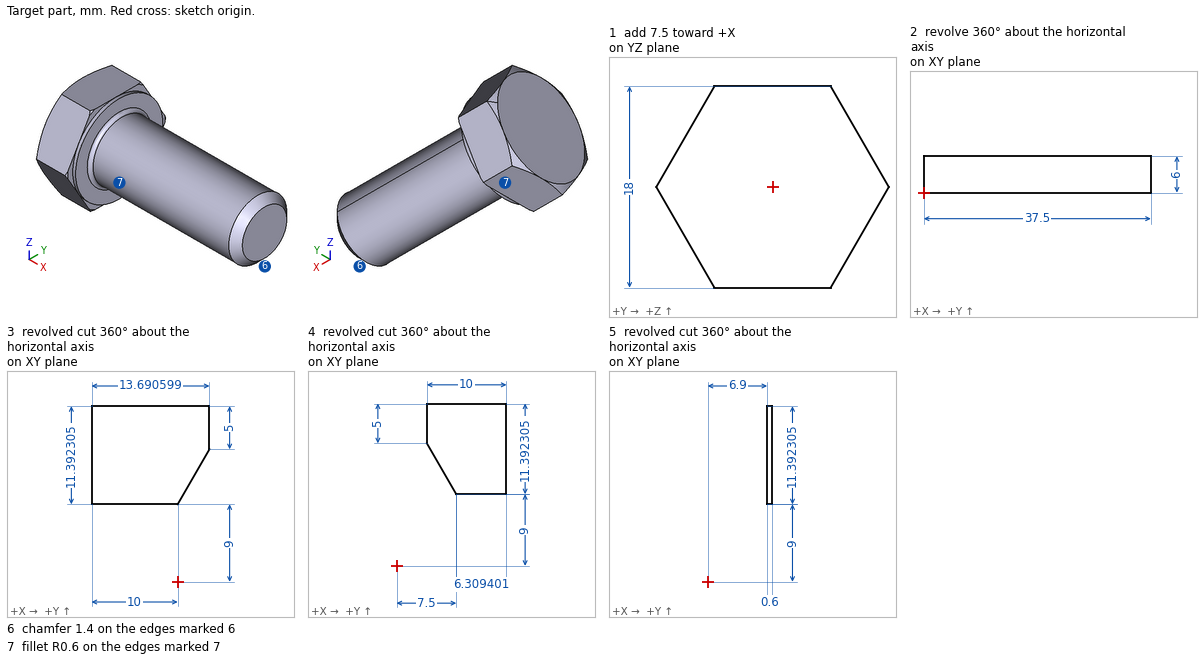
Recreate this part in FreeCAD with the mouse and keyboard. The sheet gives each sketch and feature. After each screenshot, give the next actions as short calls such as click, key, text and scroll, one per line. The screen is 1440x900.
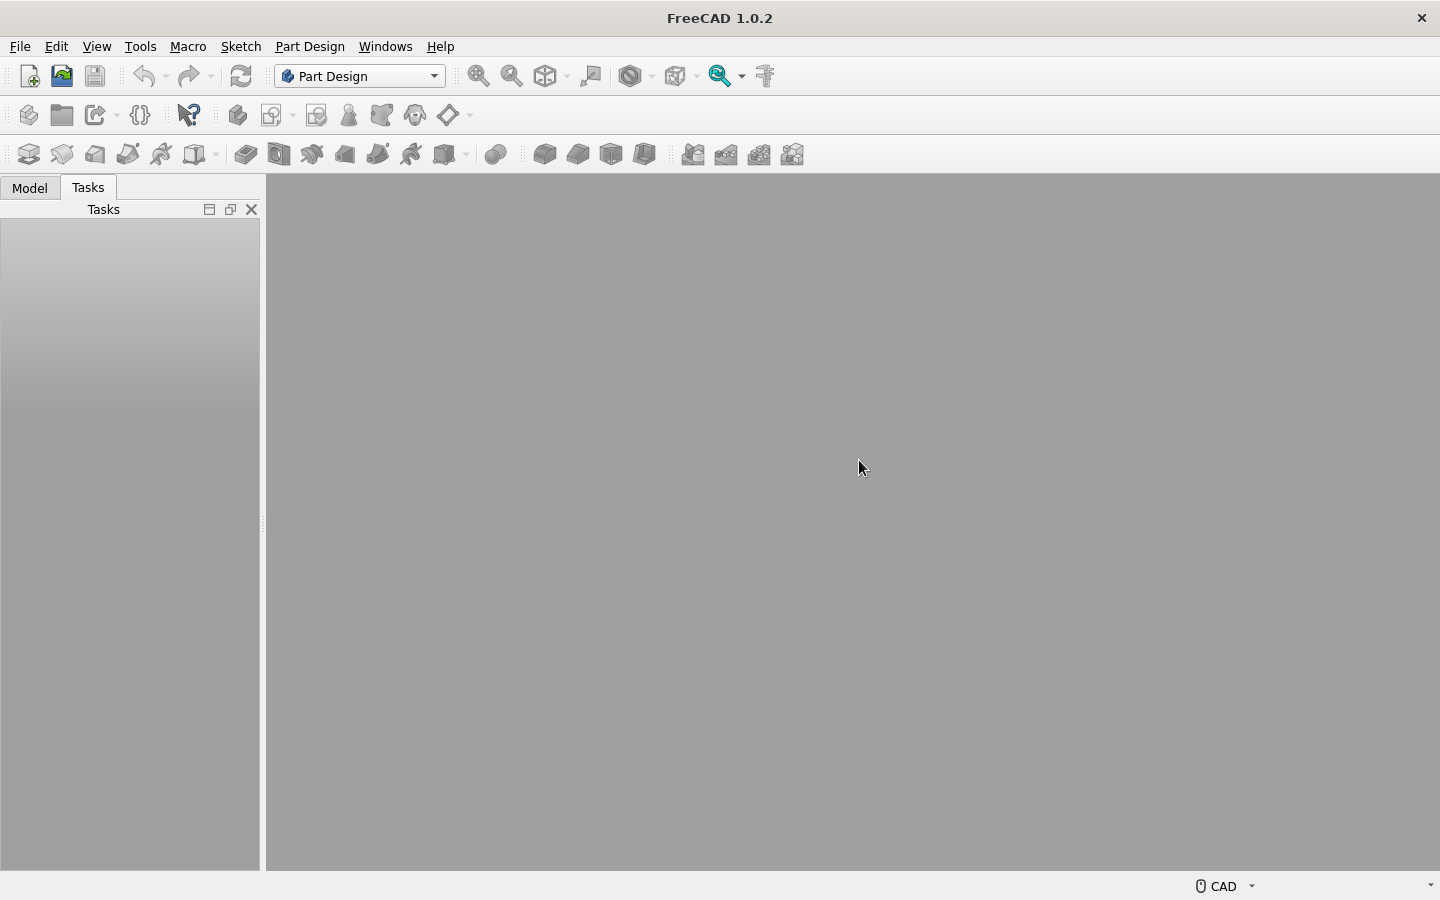
key(ctrl+n)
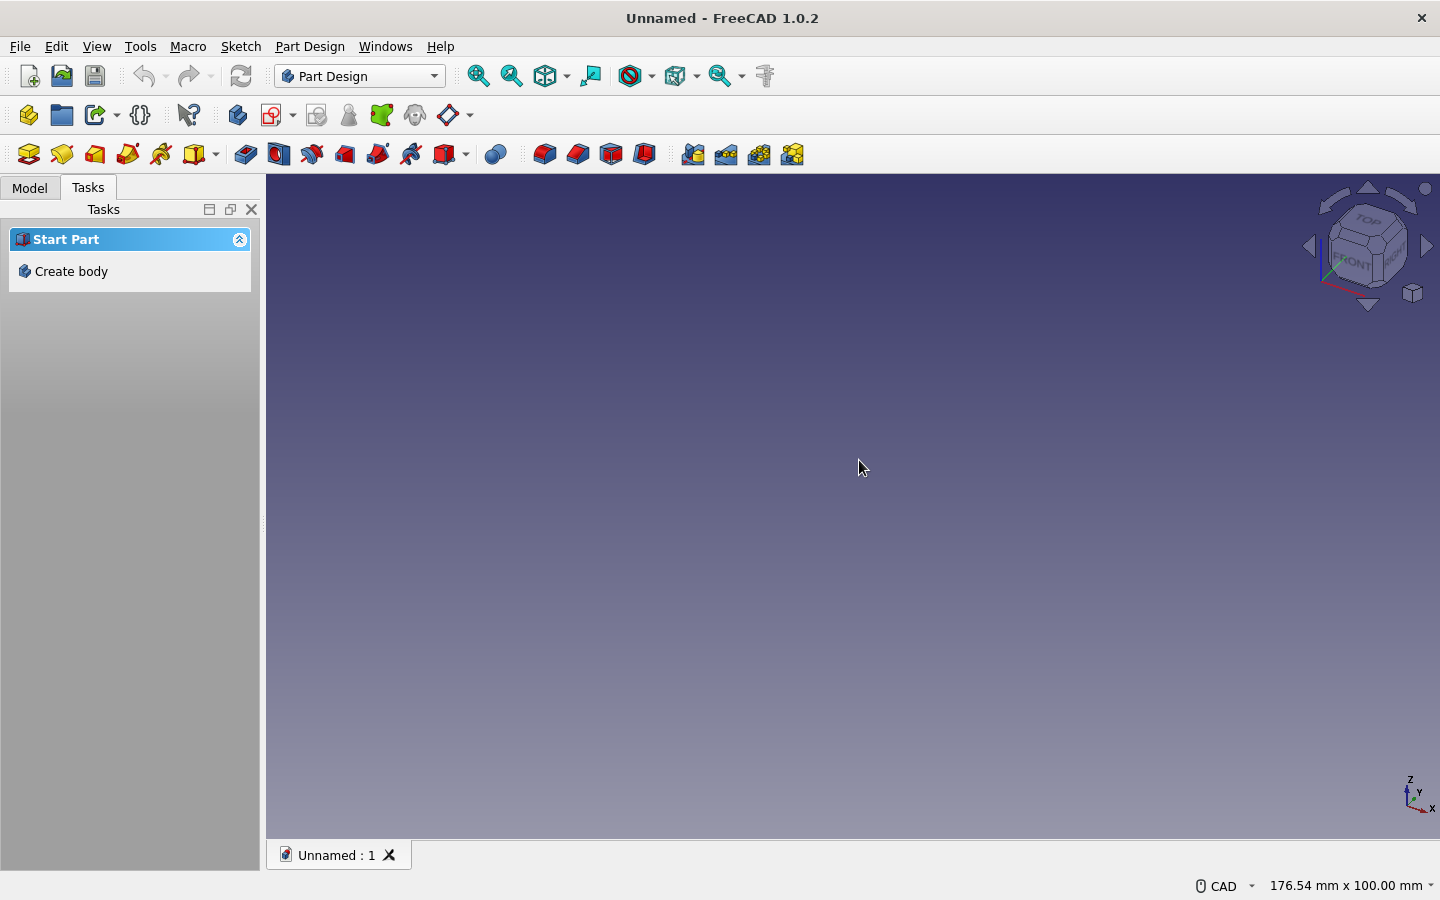
click(270, 116)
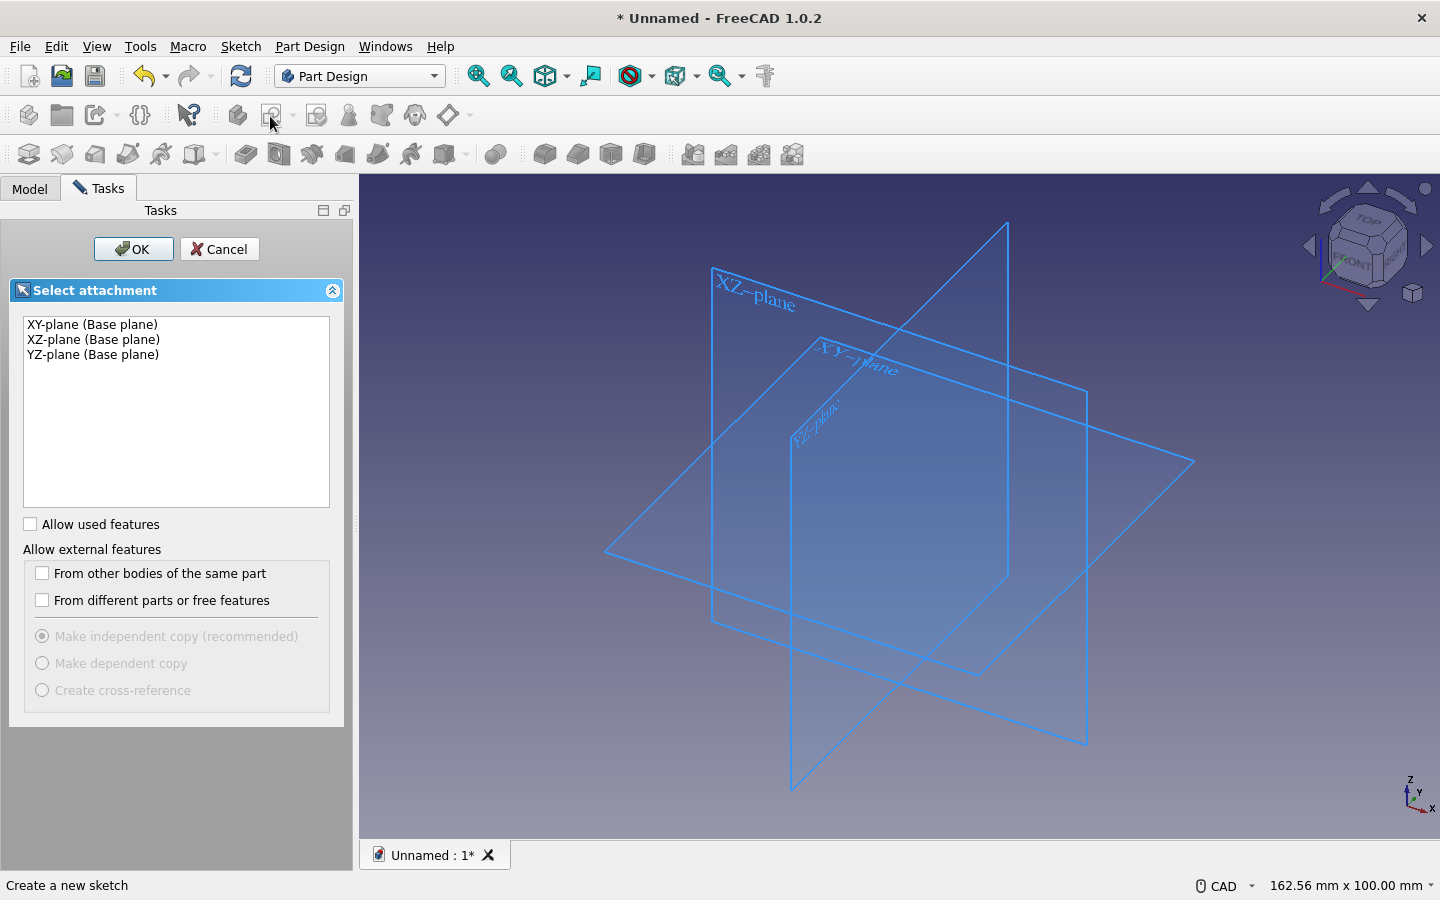
click(84, 354)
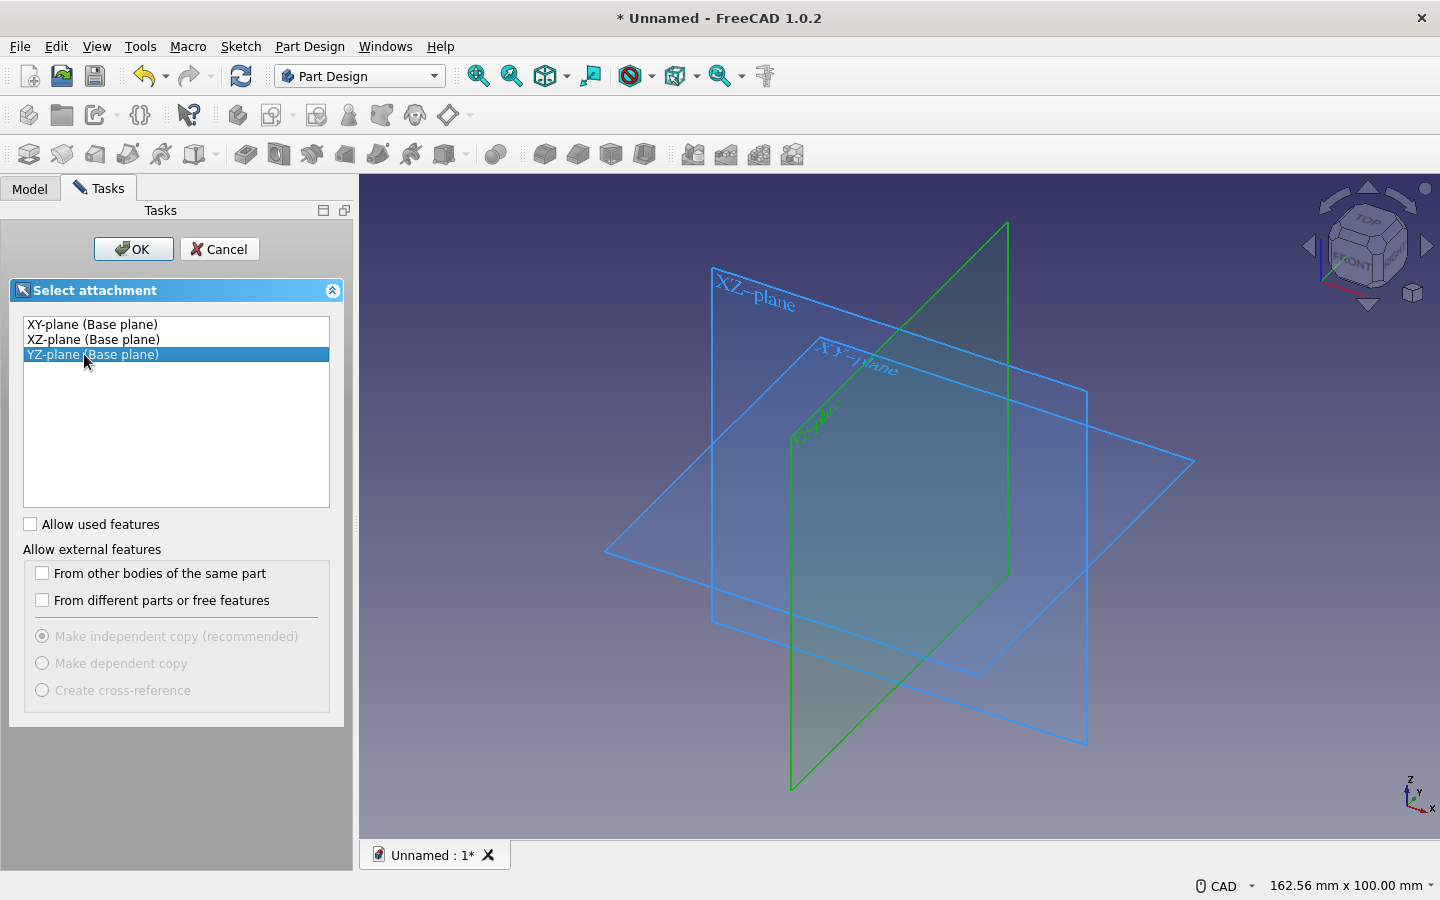
click(134, 249)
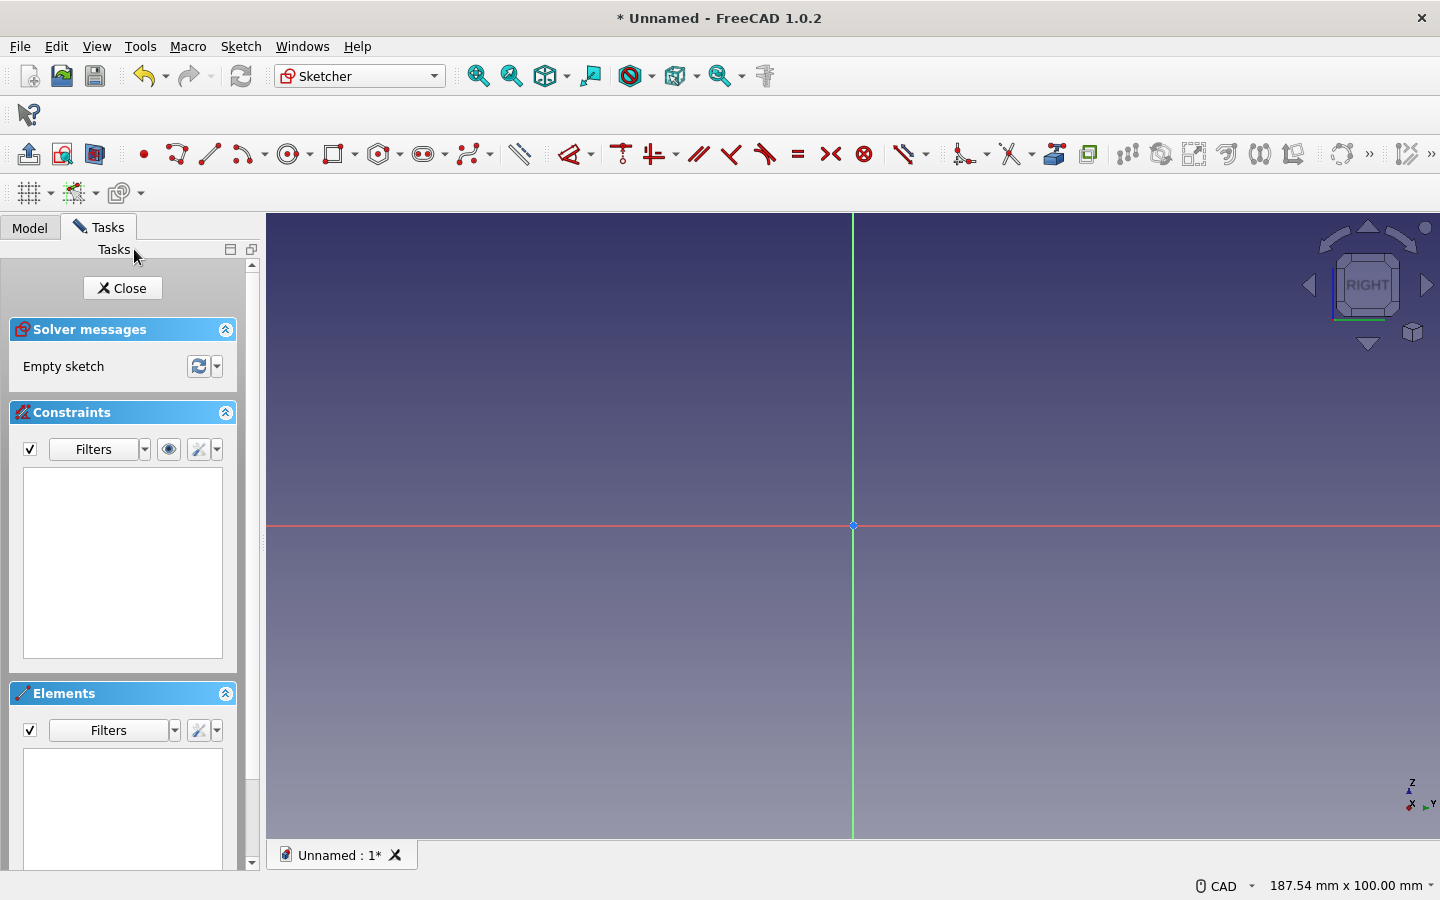
scroll(883, 526, up, 6)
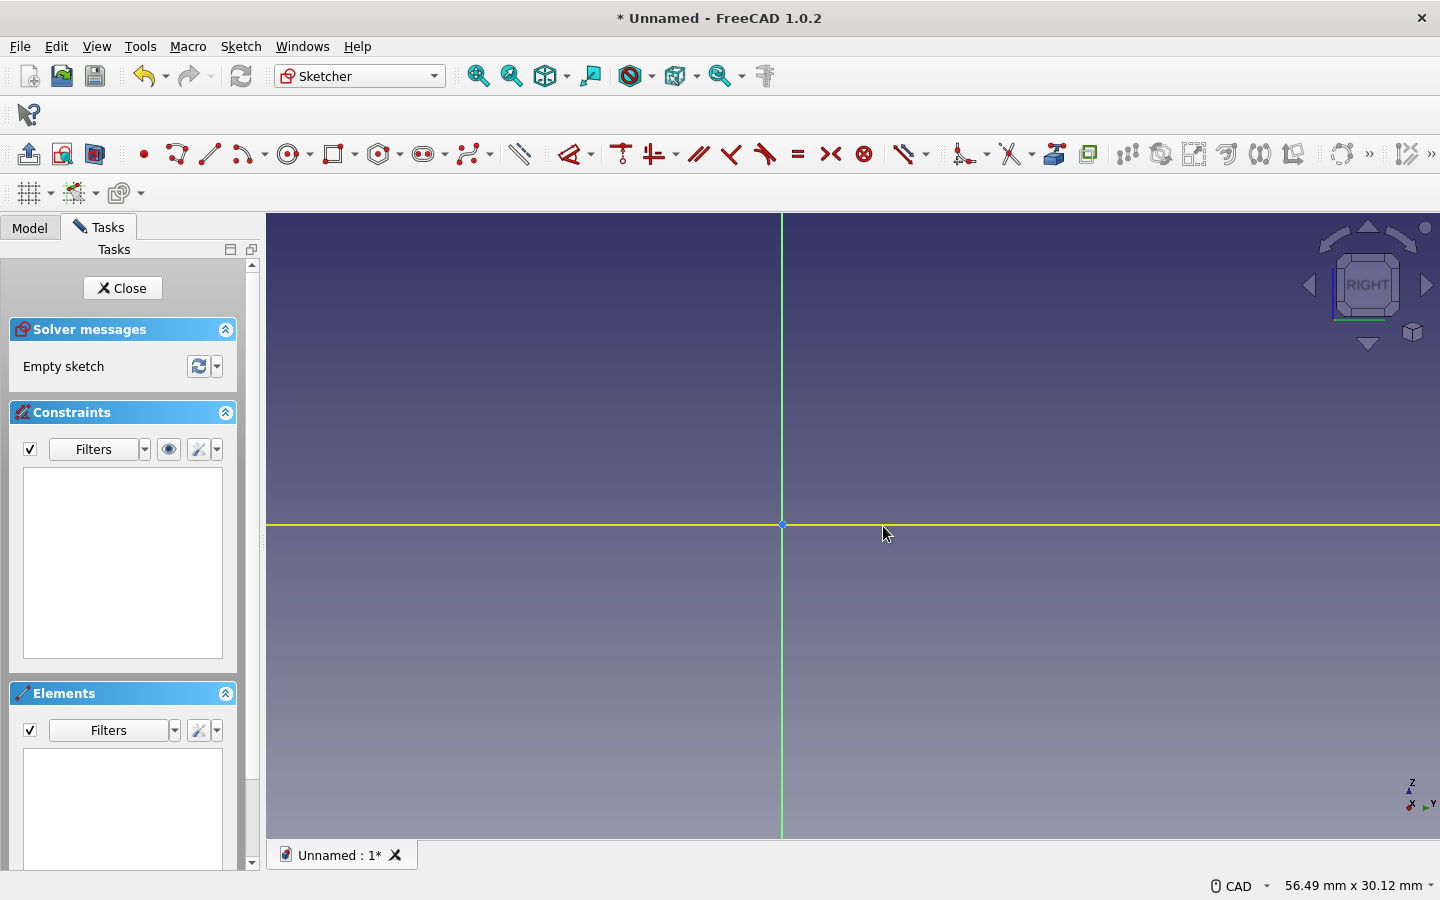
key(g)
key(p)
key(6)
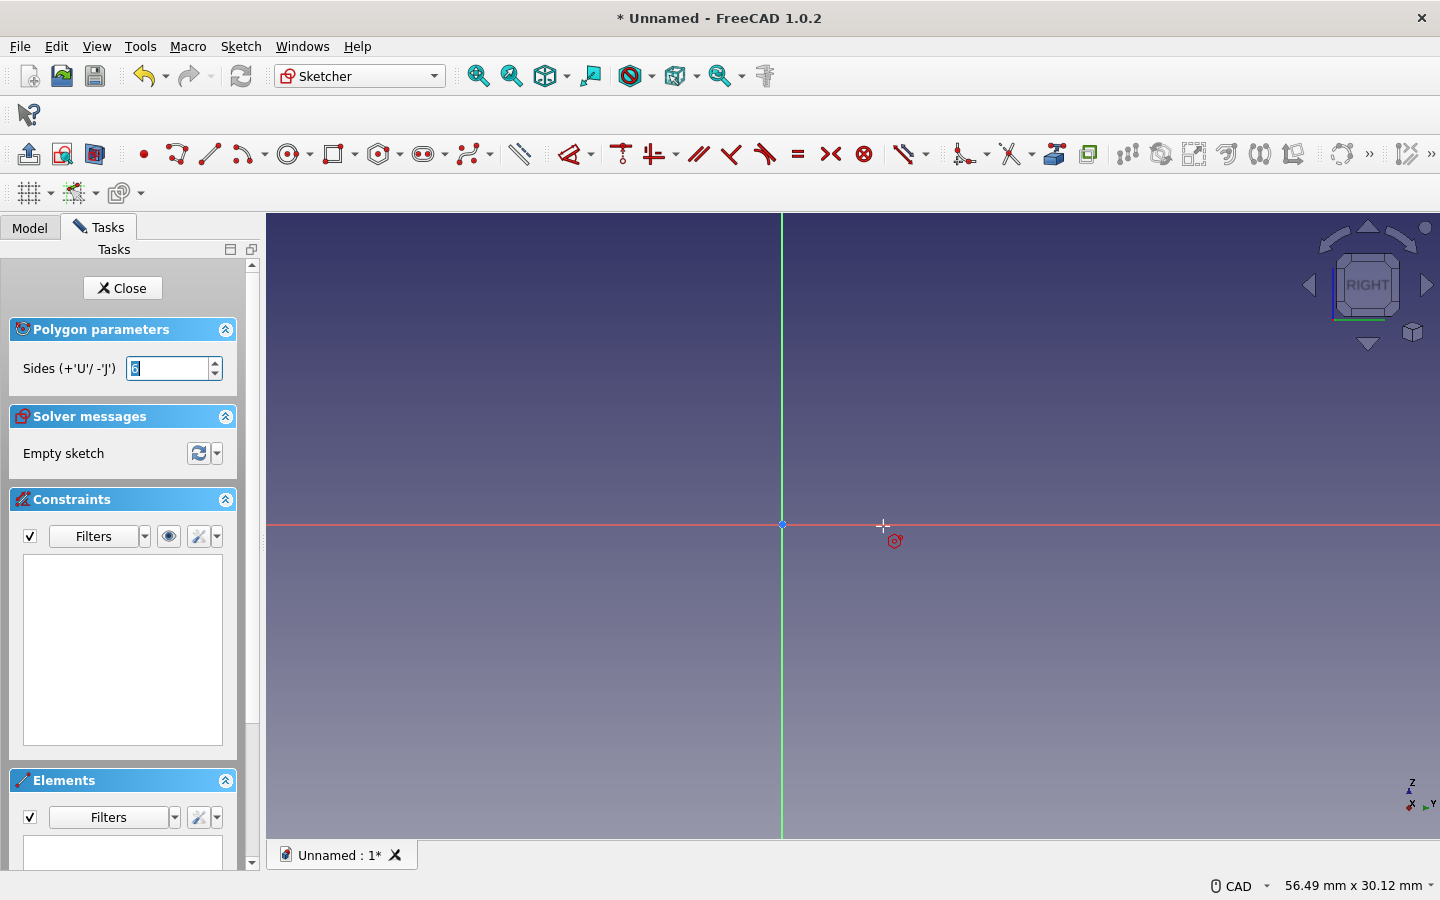
click(782, 525)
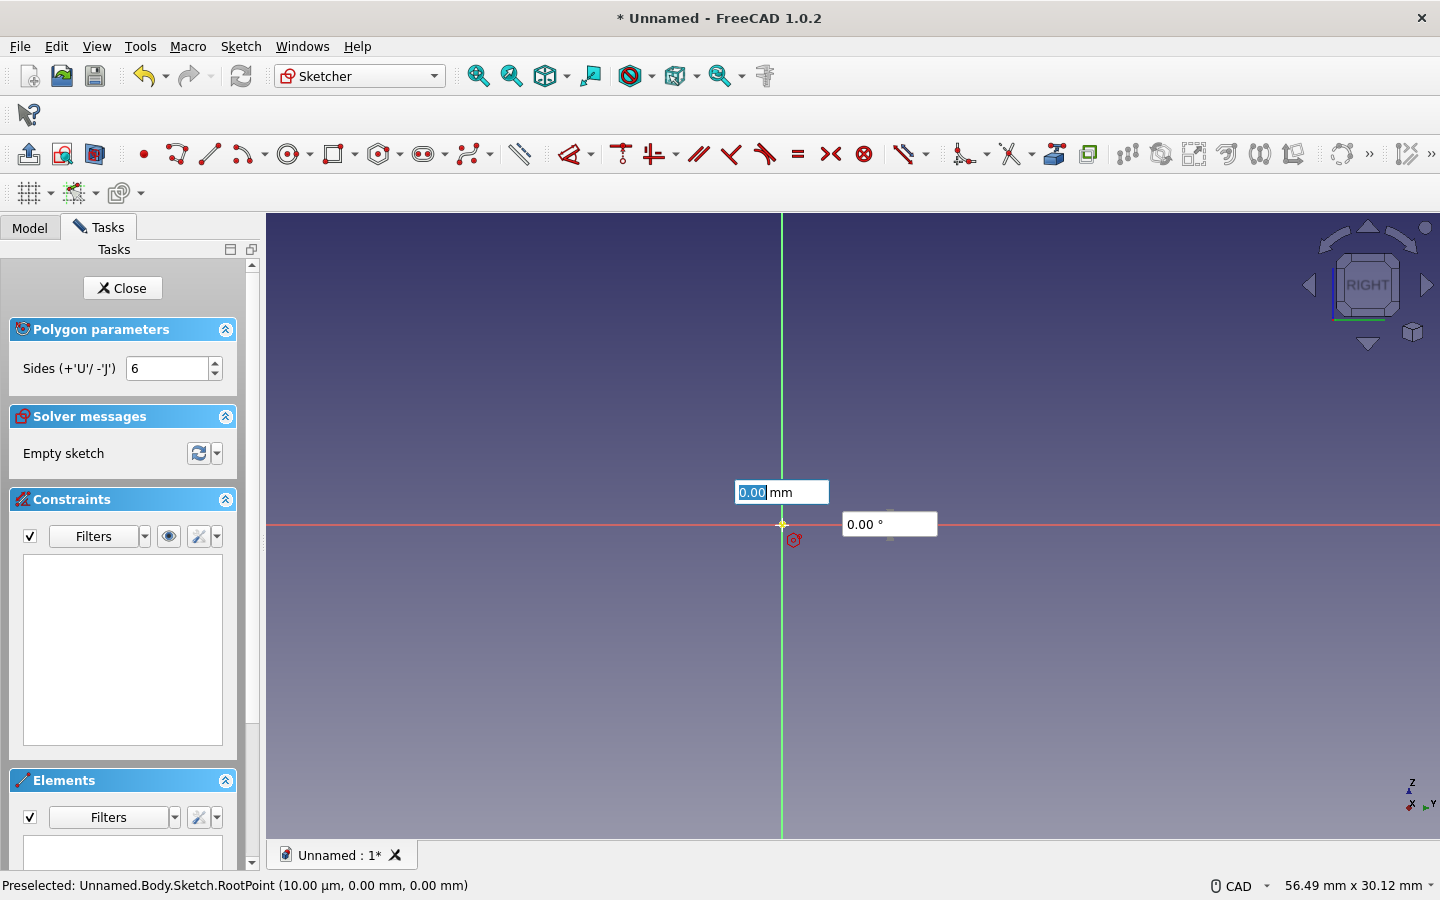
click(998, 525)
right_click(998, 525)